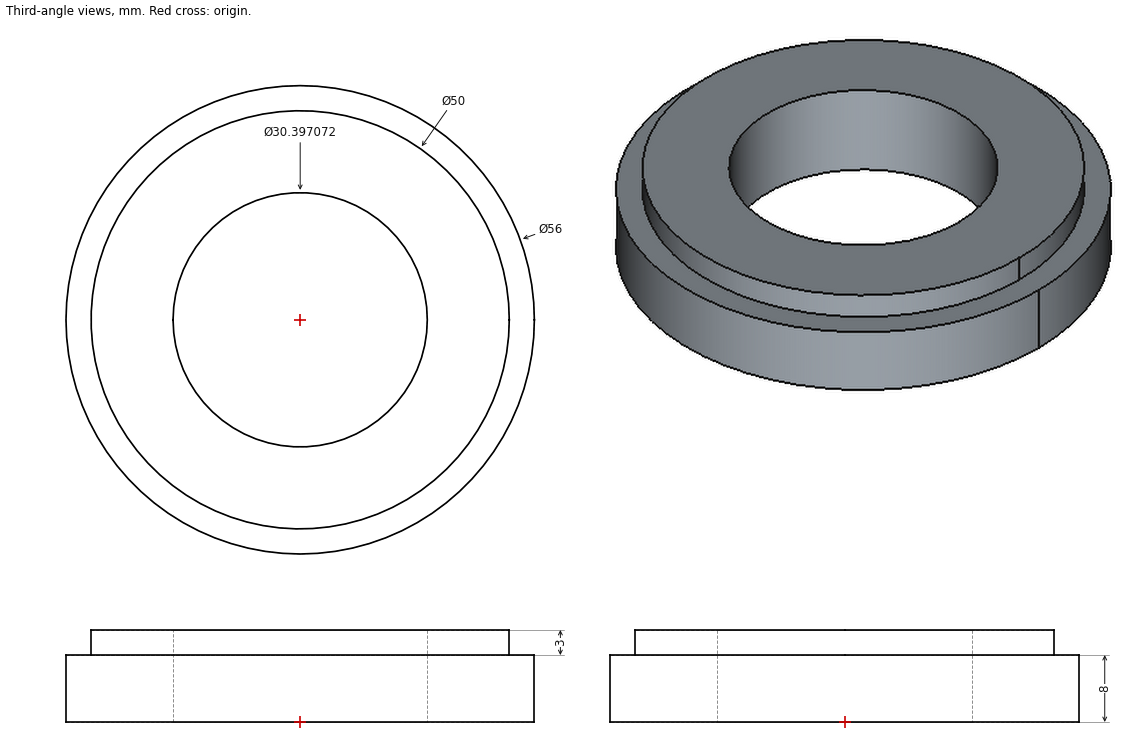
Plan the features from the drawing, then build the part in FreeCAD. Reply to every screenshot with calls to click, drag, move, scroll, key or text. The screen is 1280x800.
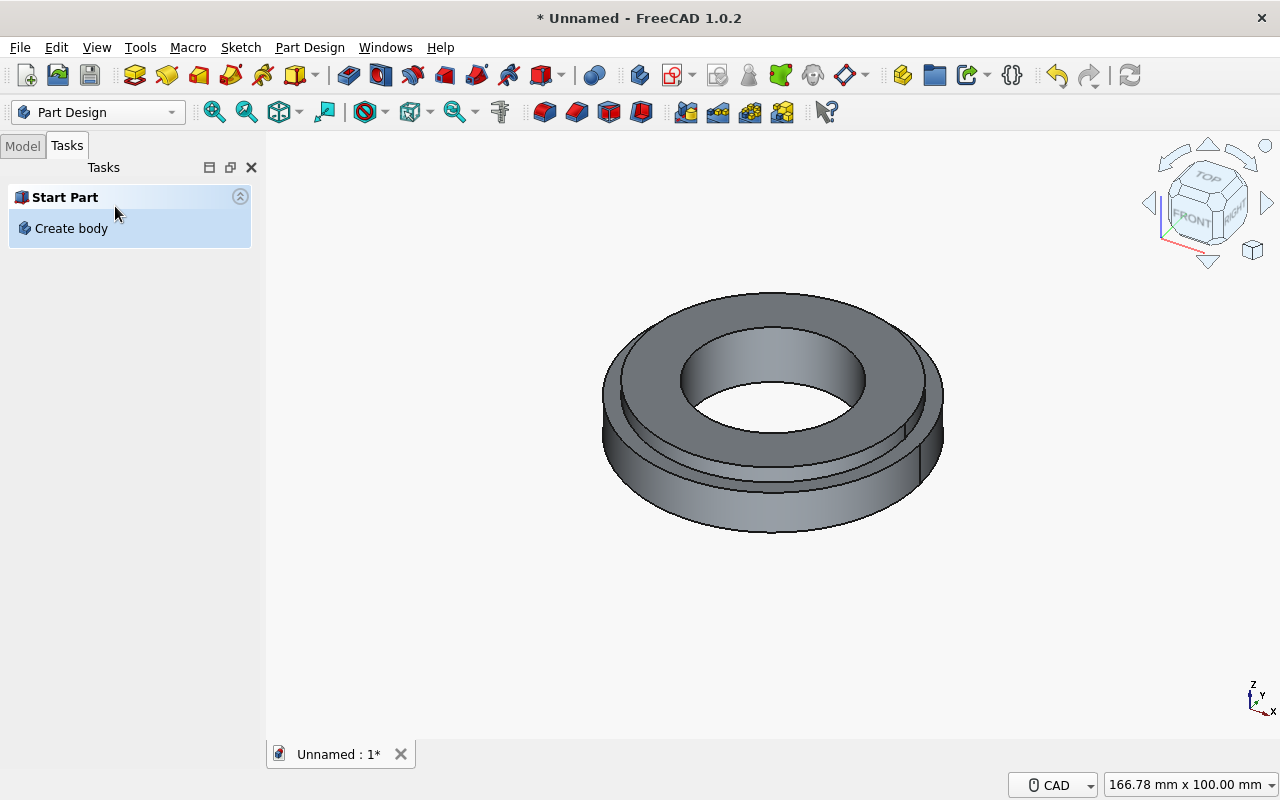
key(0)